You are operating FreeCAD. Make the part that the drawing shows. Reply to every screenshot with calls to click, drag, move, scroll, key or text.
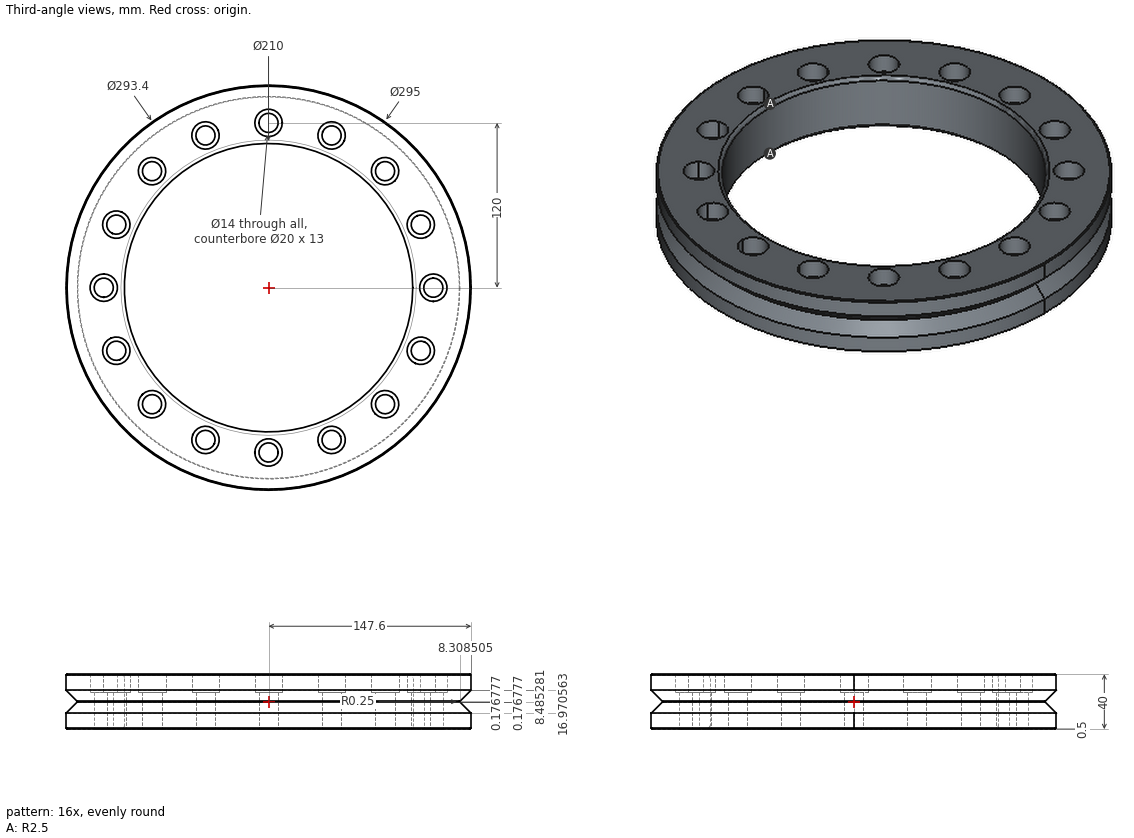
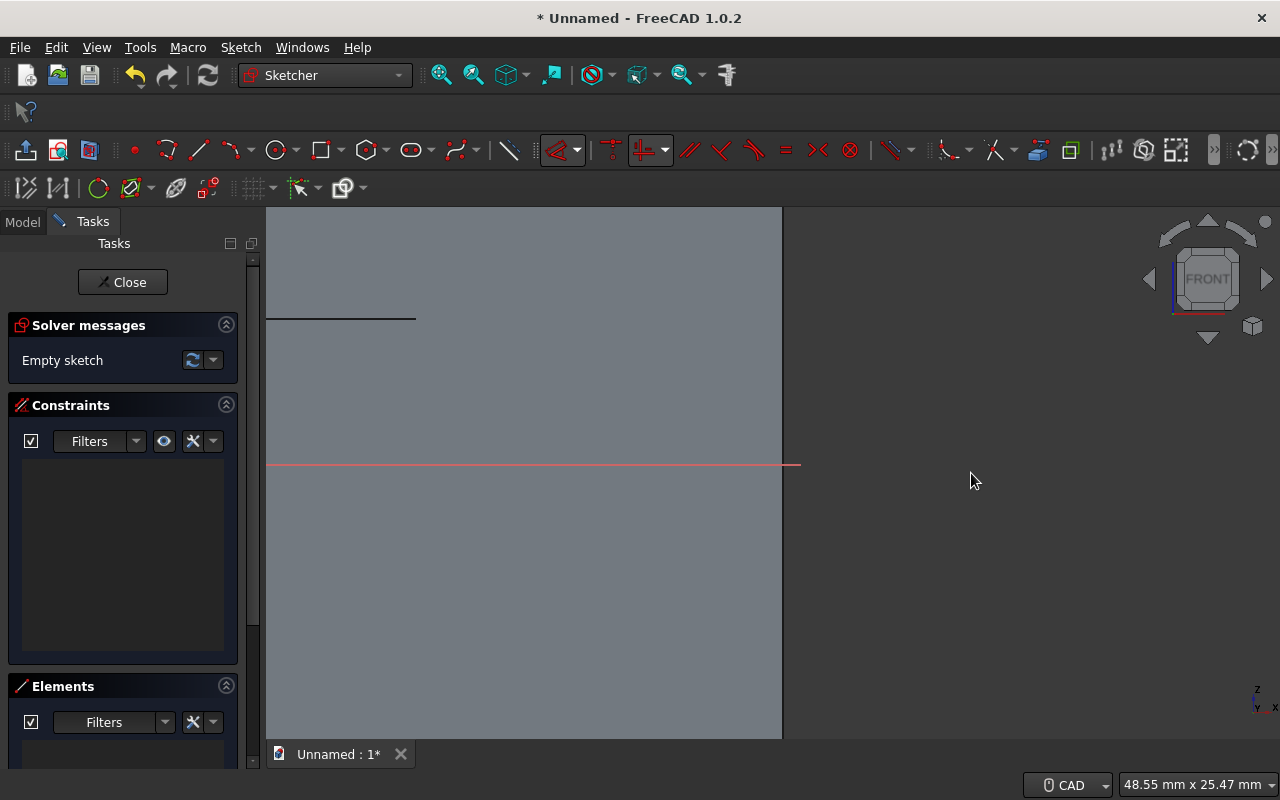
key(g)
key(m)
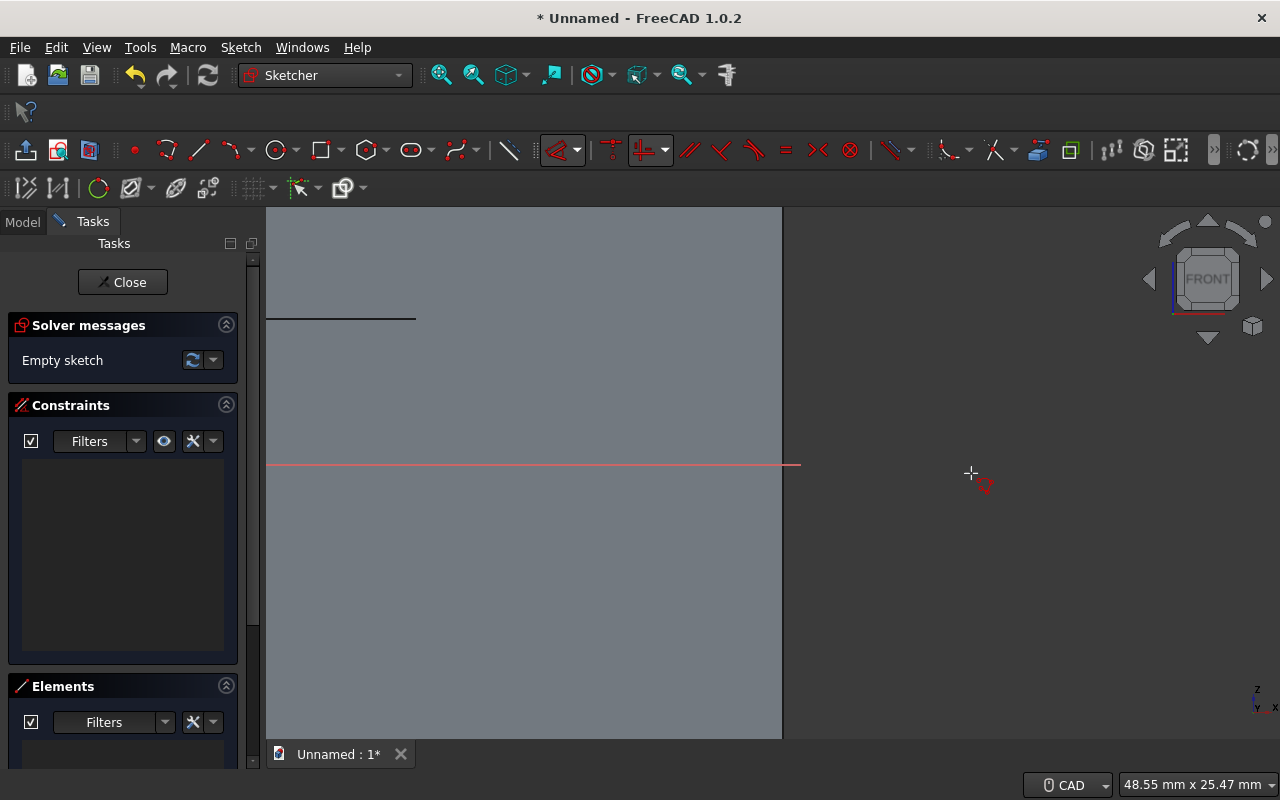
scroll(611, 462, up, 8)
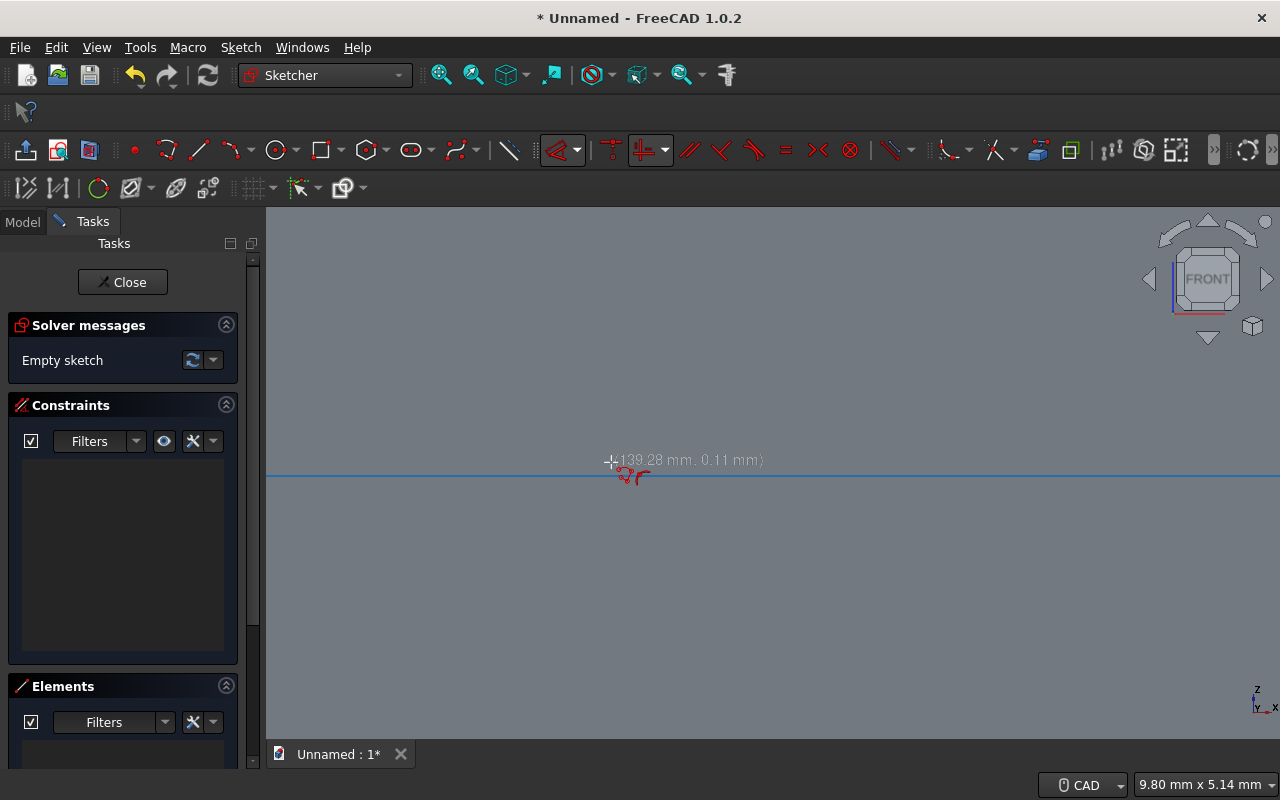
click(611, 458)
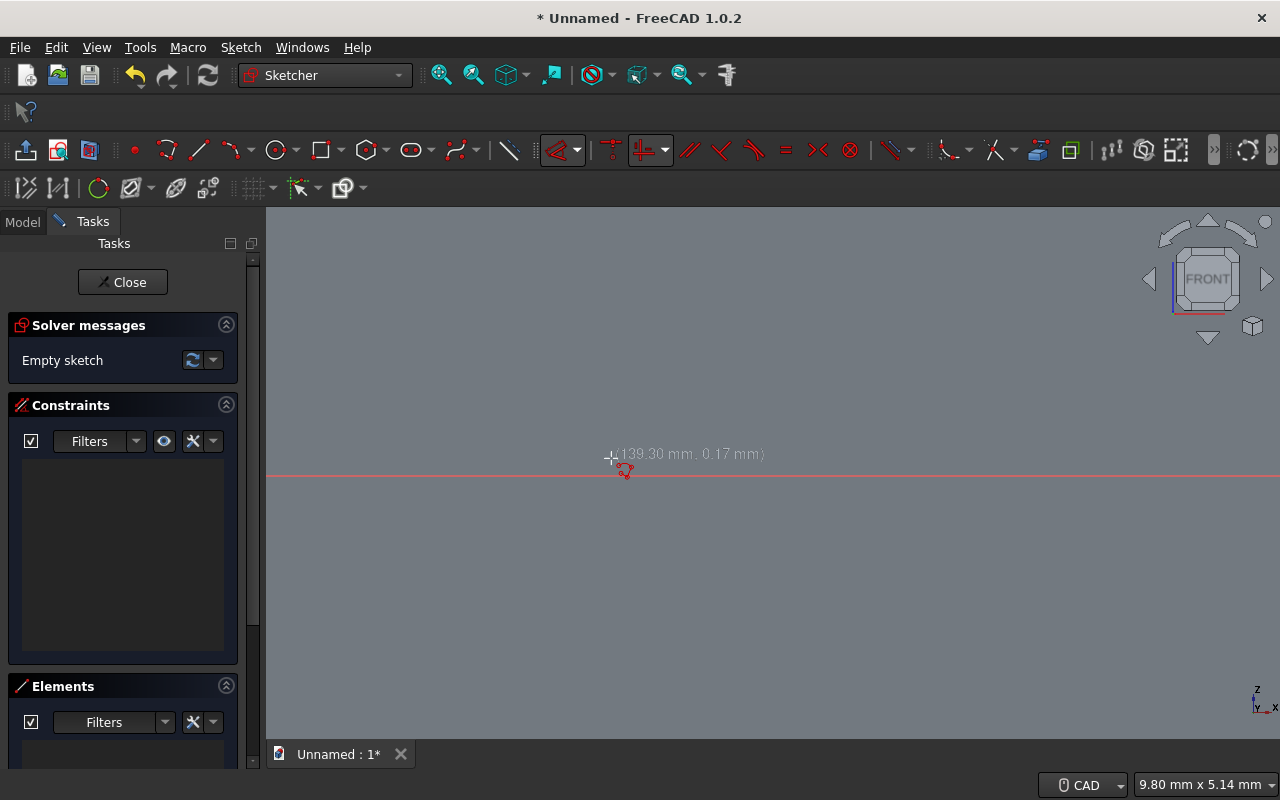
scroll(625, 472, down, 8)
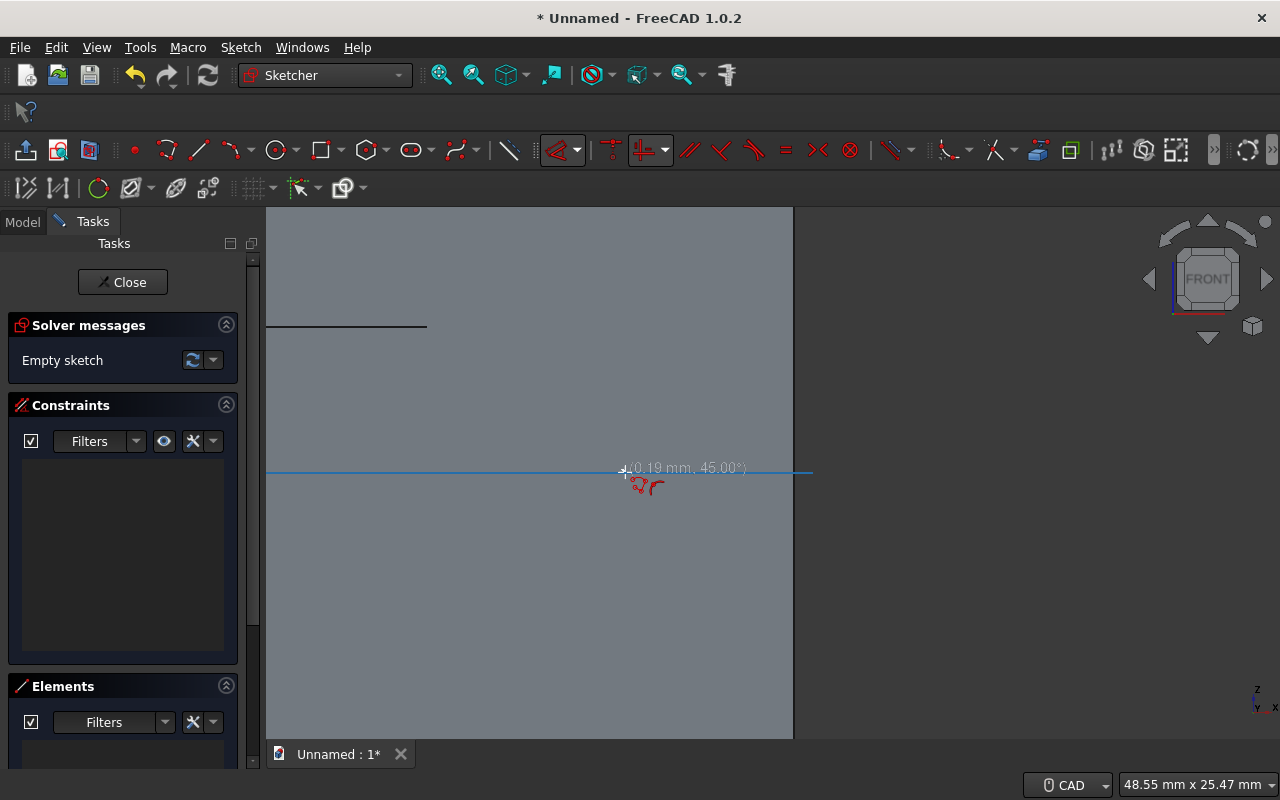
click(796, 296)
click(796, 650)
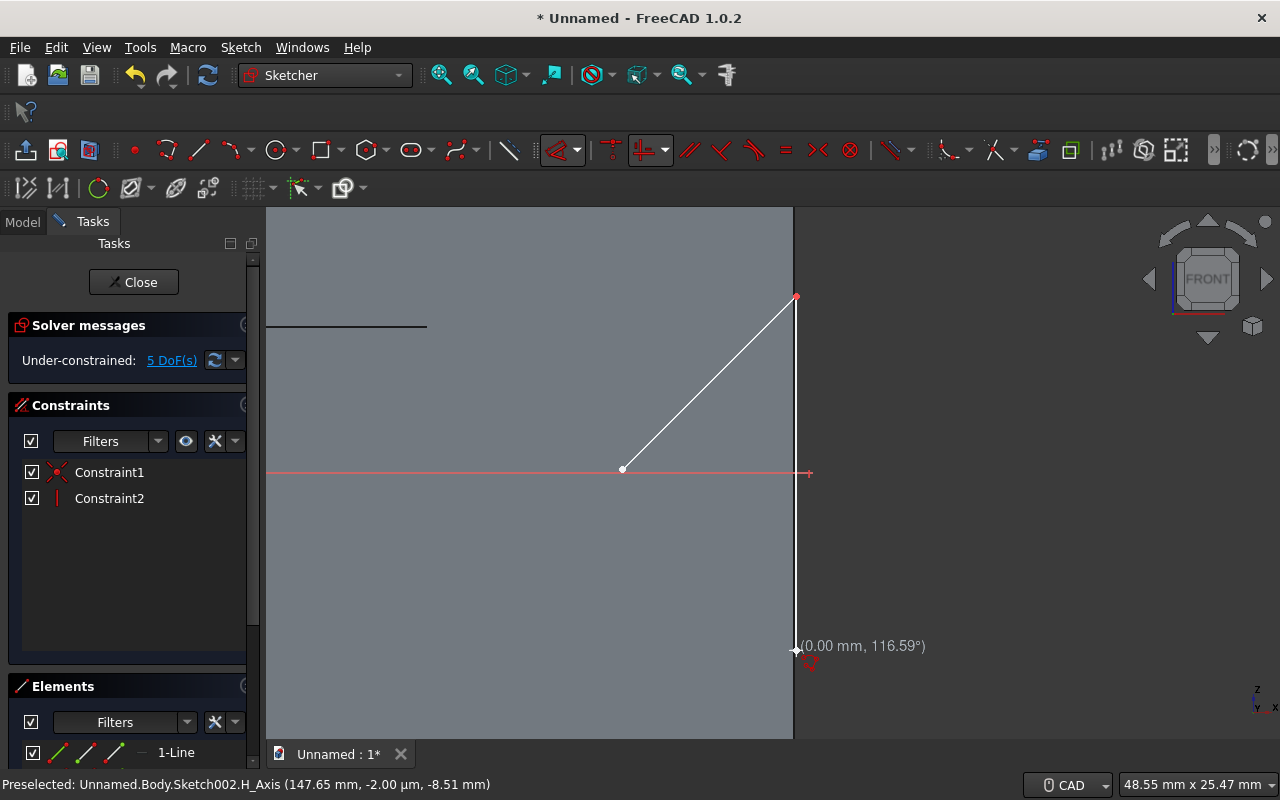
scroll(622, 477, up, 8)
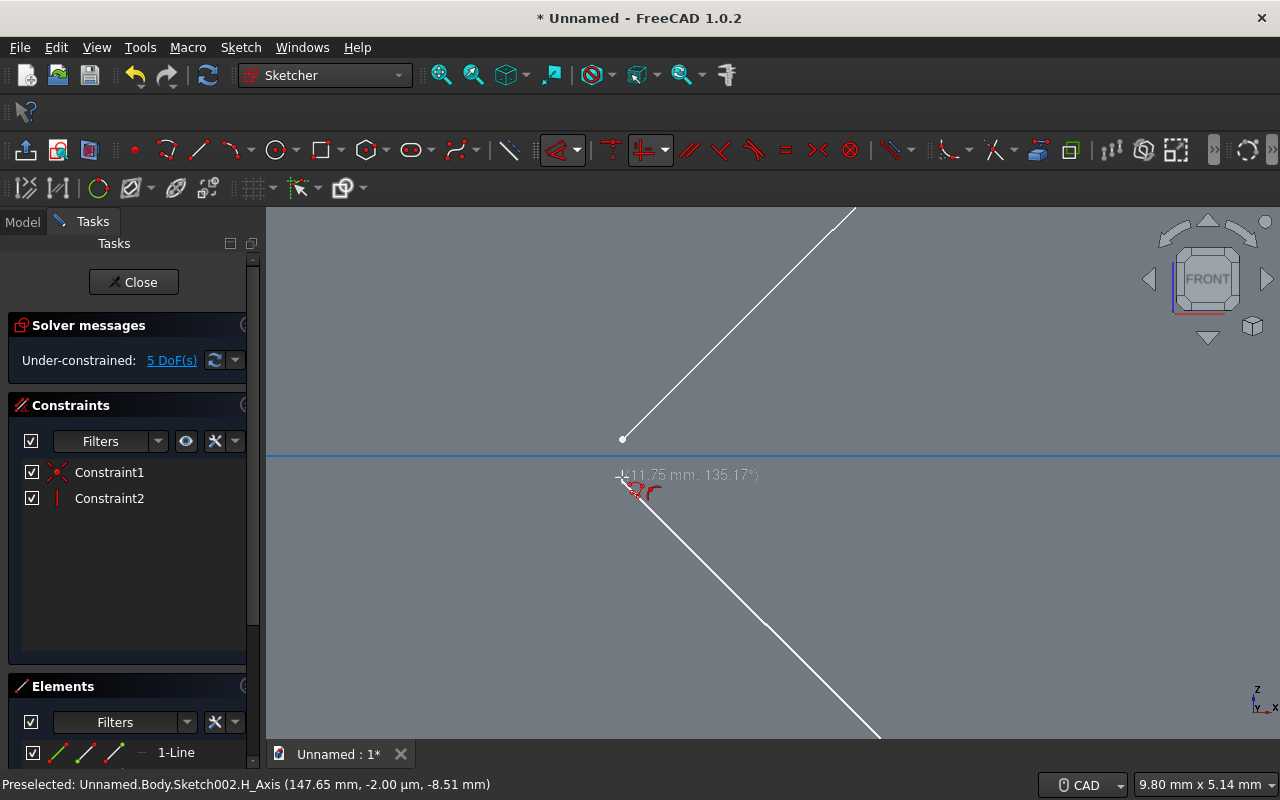
click(622, 475)
right_click(622, 475)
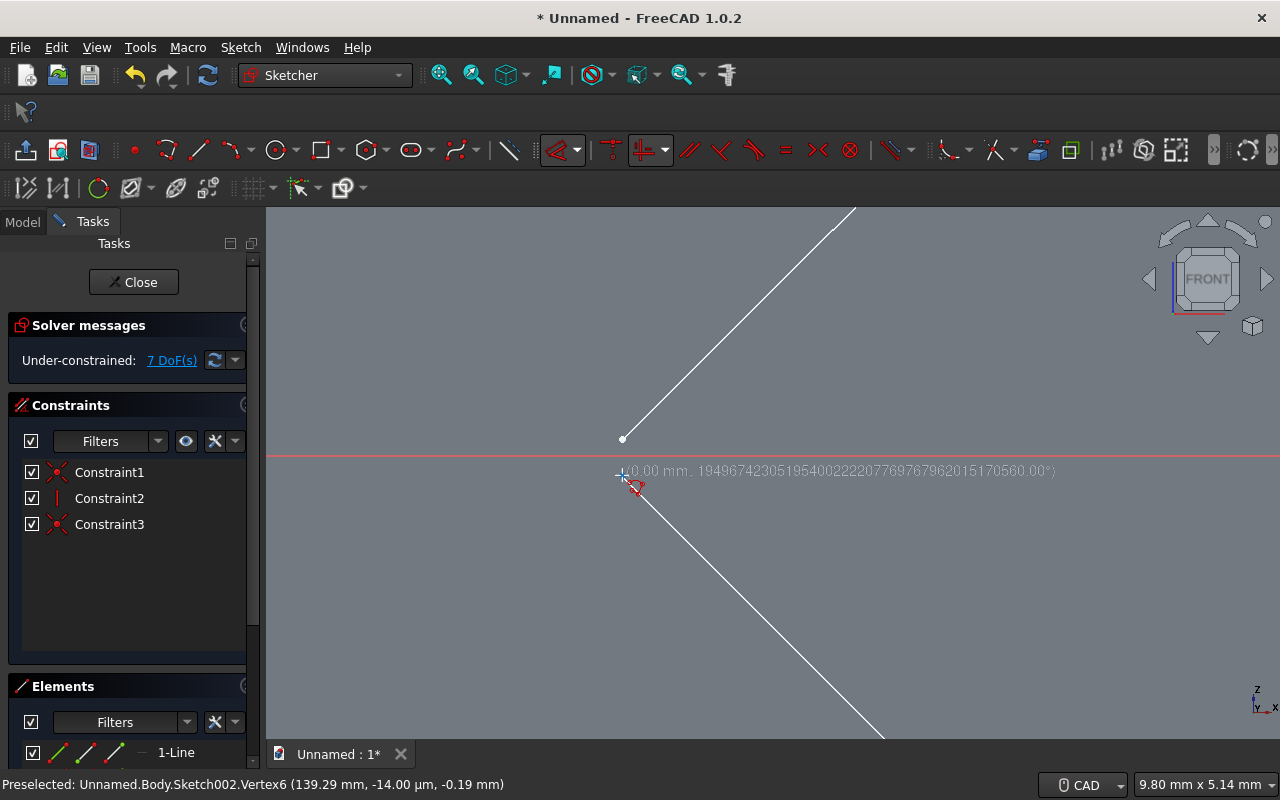
key(g)
key(3)
key(a)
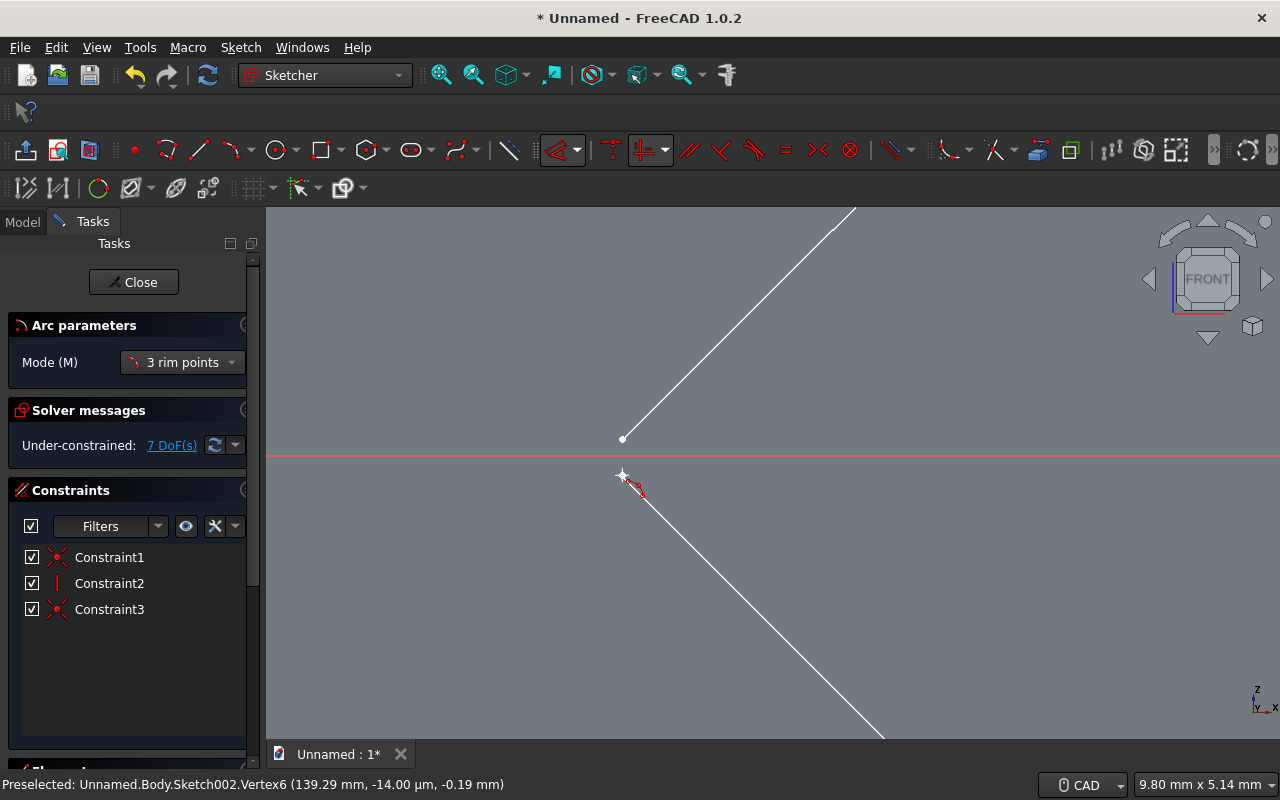
click(622, 476)
click(623, 439)
click(589, 436)
key(Escape)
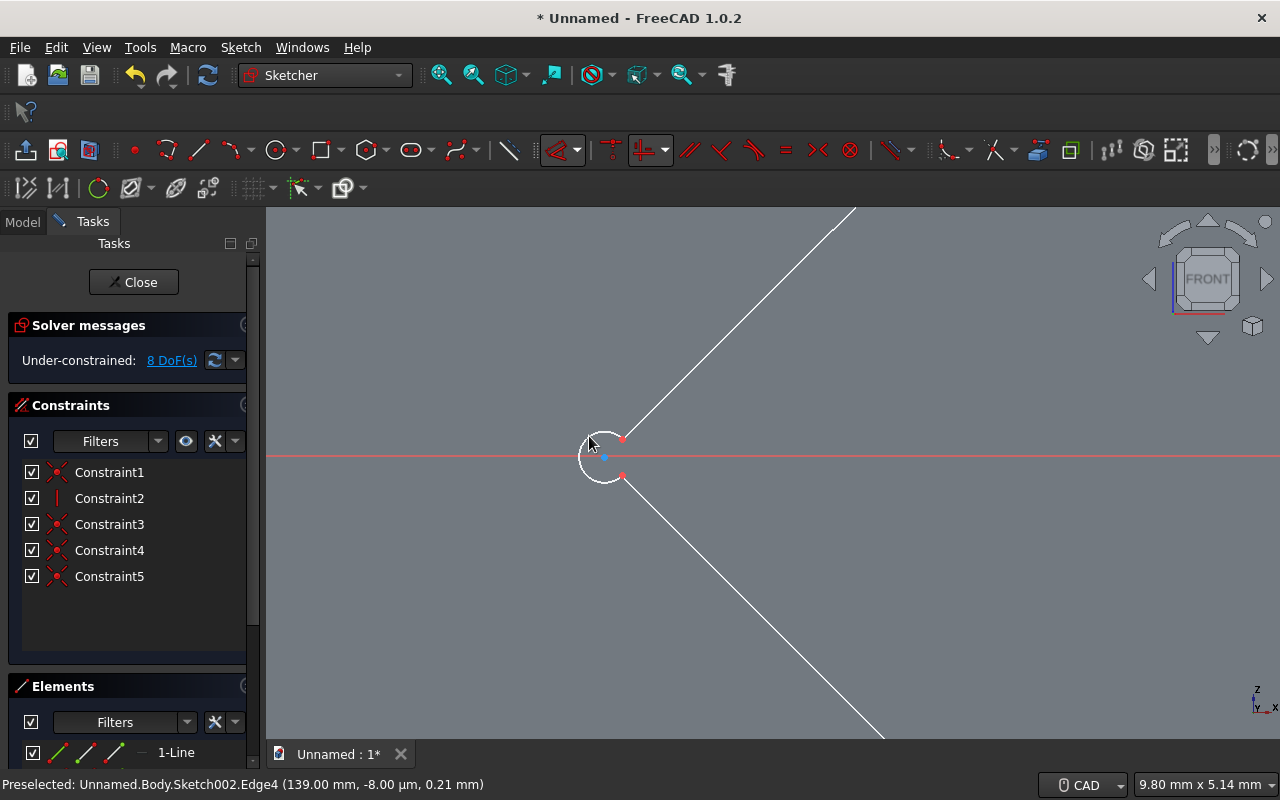
click(605, 457)